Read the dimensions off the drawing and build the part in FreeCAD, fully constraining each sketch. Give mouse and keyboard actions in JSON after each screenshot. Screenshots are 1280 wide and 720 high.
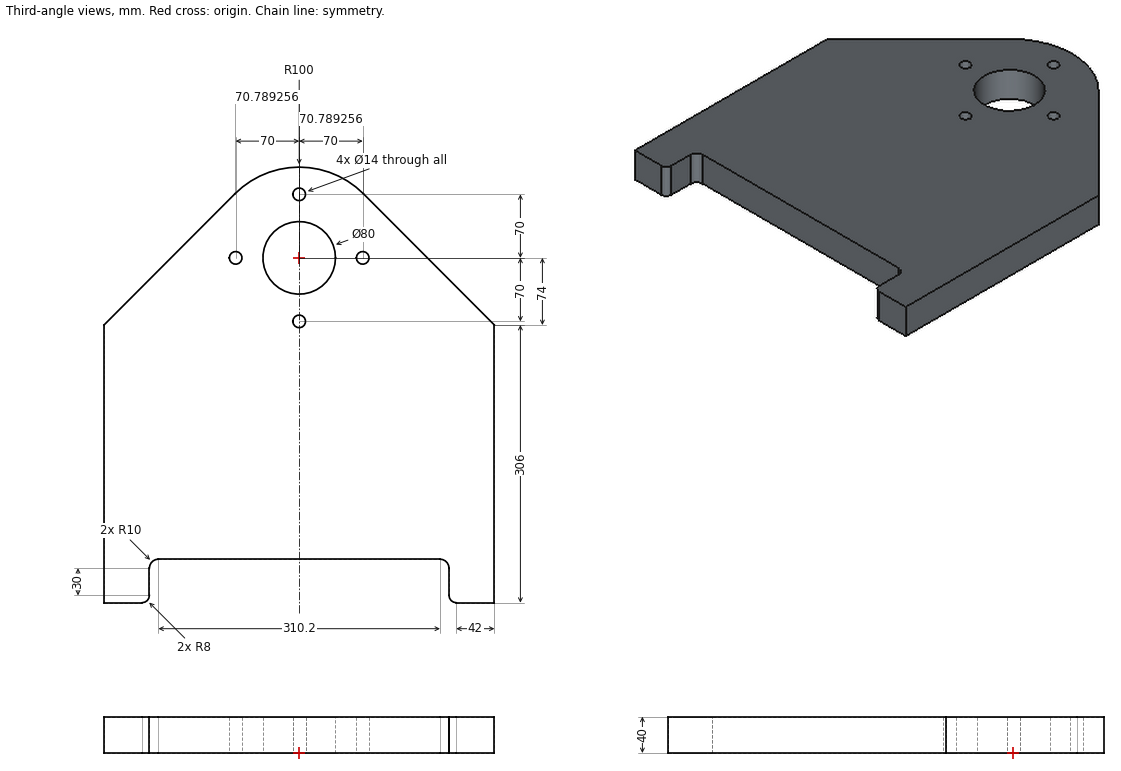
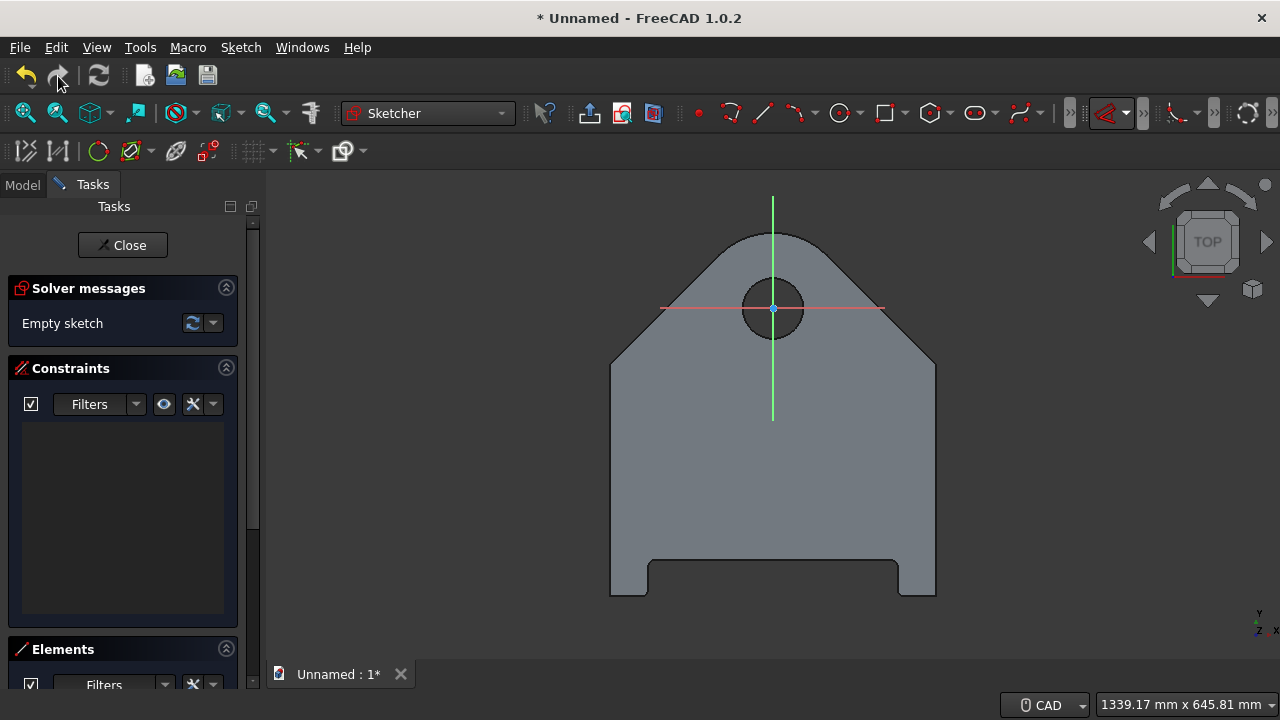
{"action": "scroll", "coordinate": [813, 247], "scroll_direction": "up", "scroll_amount": 5}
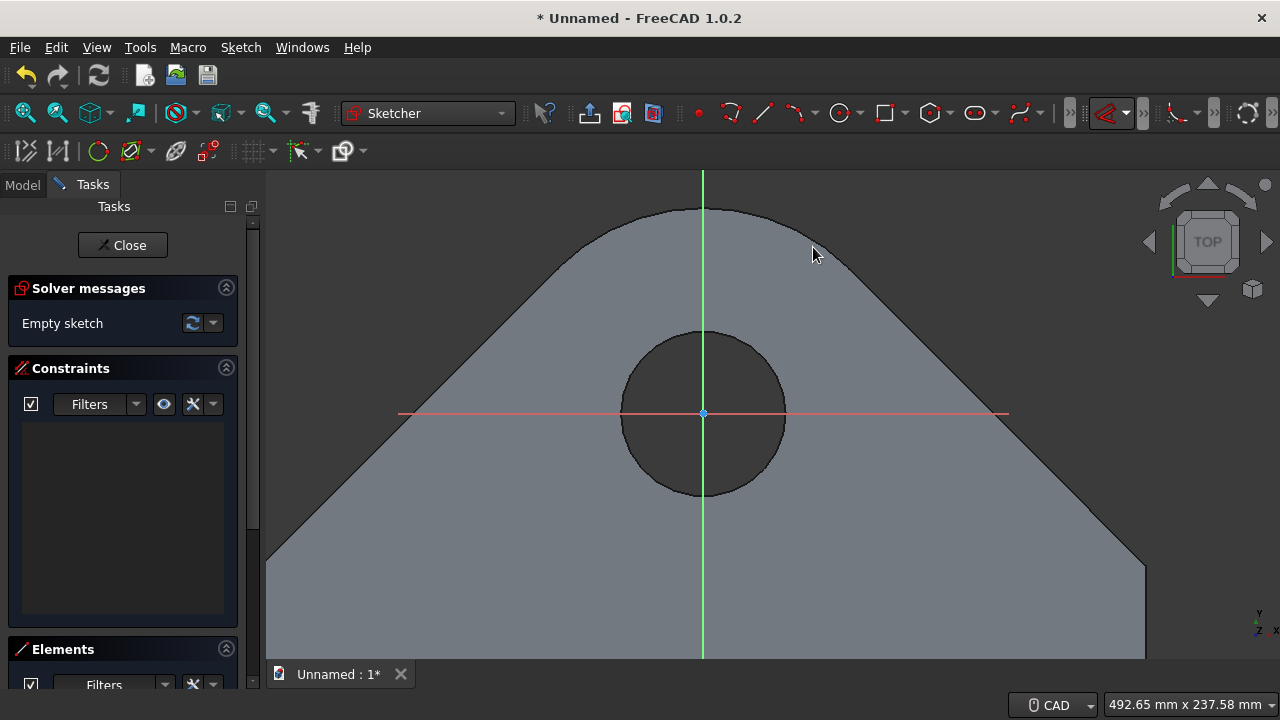
{"action": "key", "text": "g c"}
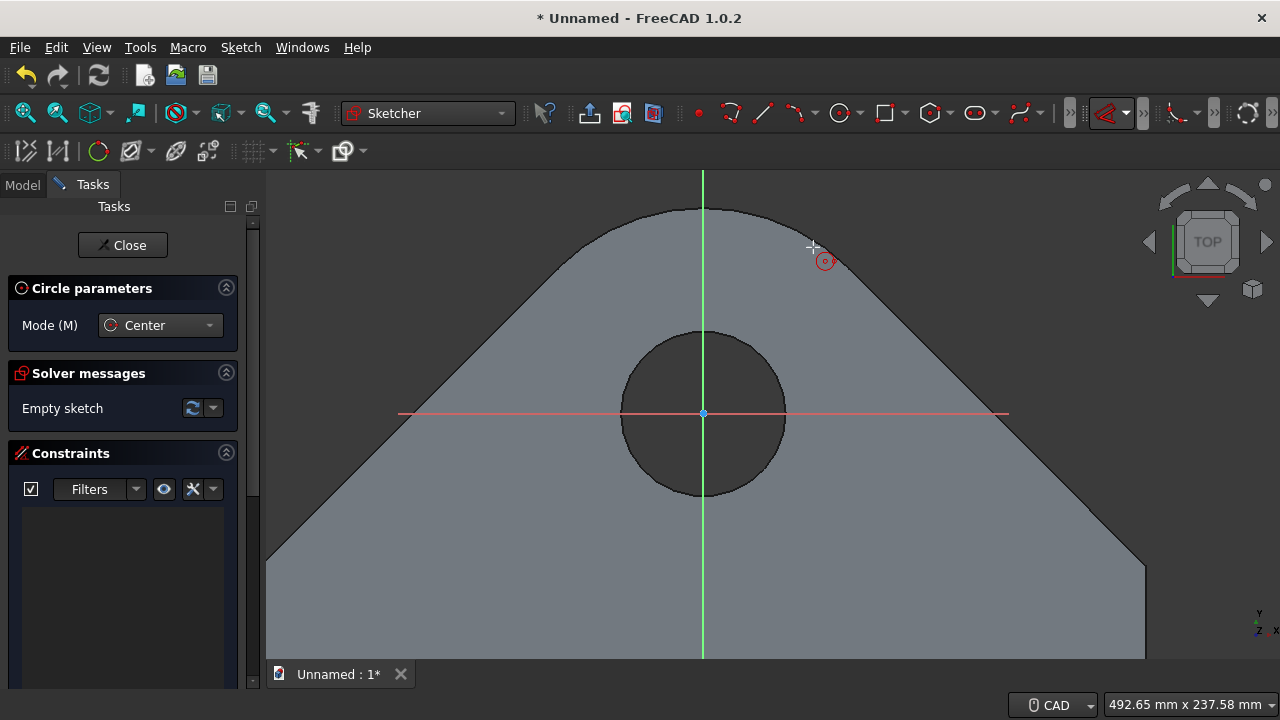
{"action": "scroll", "coordinate": [703, 270], "scroll_direction": "up", "scroll_amount": 3}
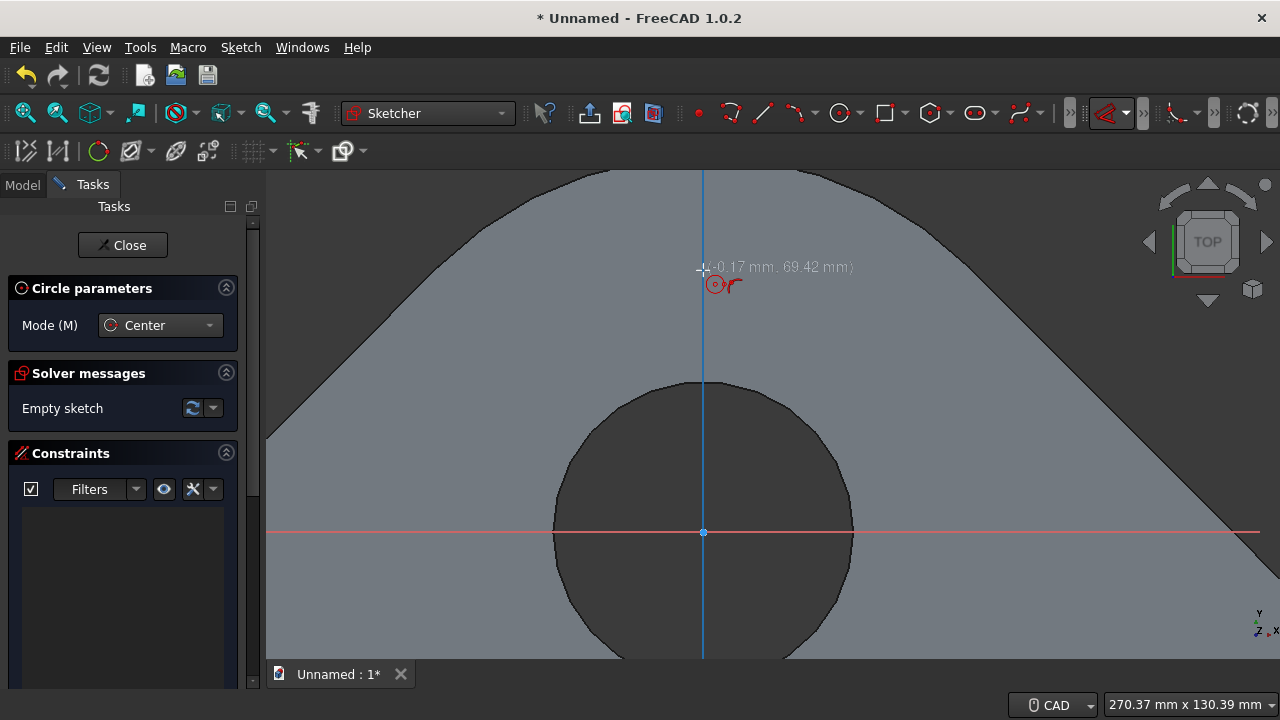
{"action": "left_click", "coordinate": [703, 269]}
{"action": "left_click", "coordinate": [722, 251]}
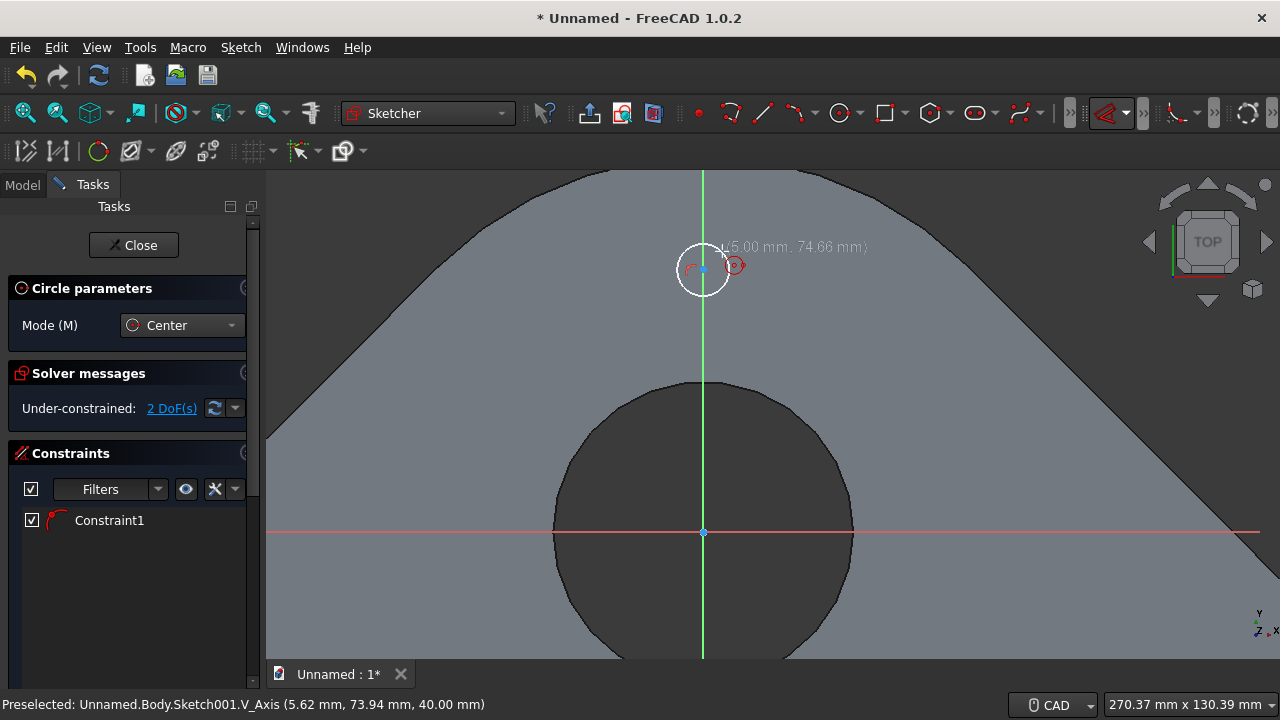
{"action": "left_click", "coordinate": [966, 532]}
{"action": "left_click", "coordinate": [984, 513]}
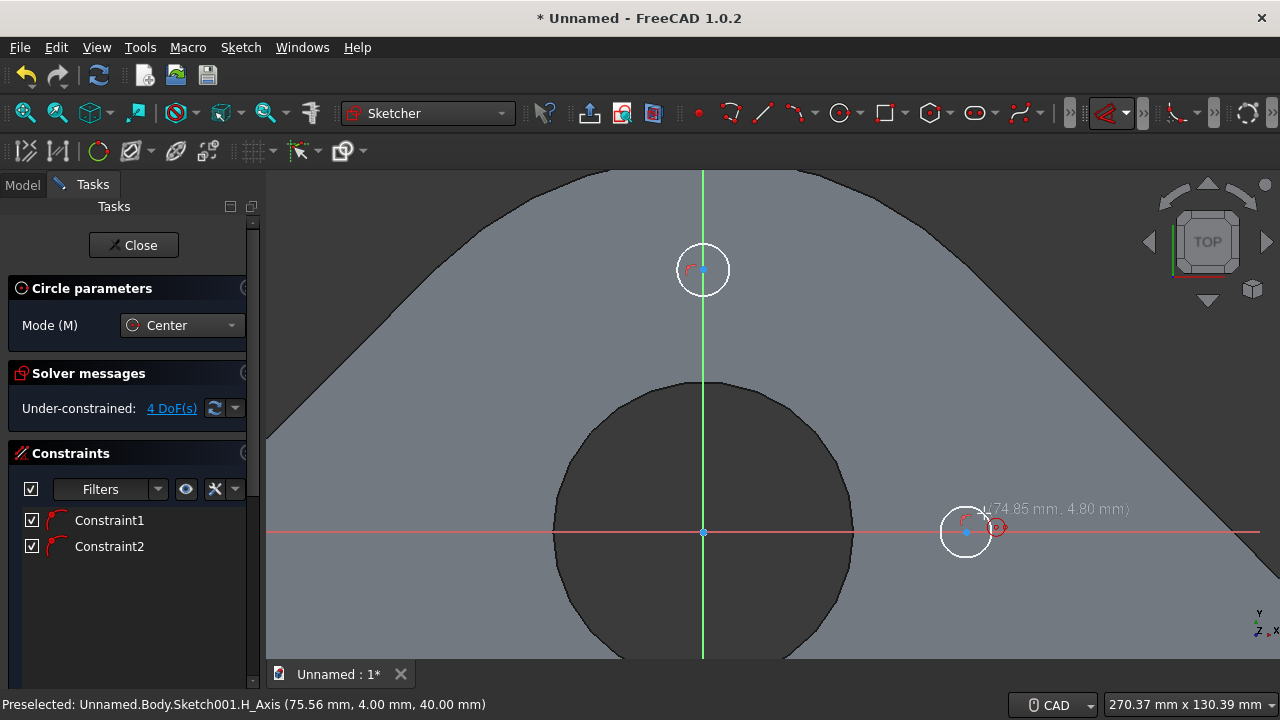
{"action": "scroll", "coordinate": [706, 272], "scroll_direction": "down", "scroll_amount": 3}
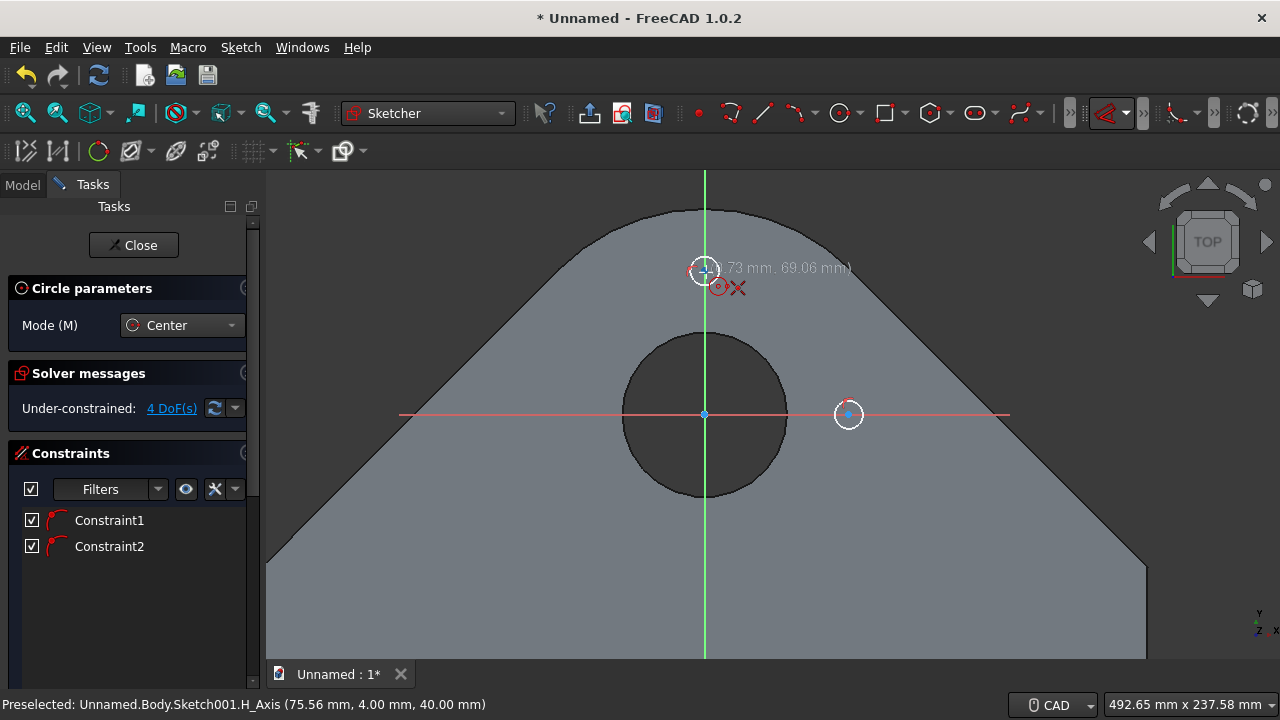
{"action": "scroll", "coordinate": [705, 559], "scroll_direction": "up", "scroll_amount": 3}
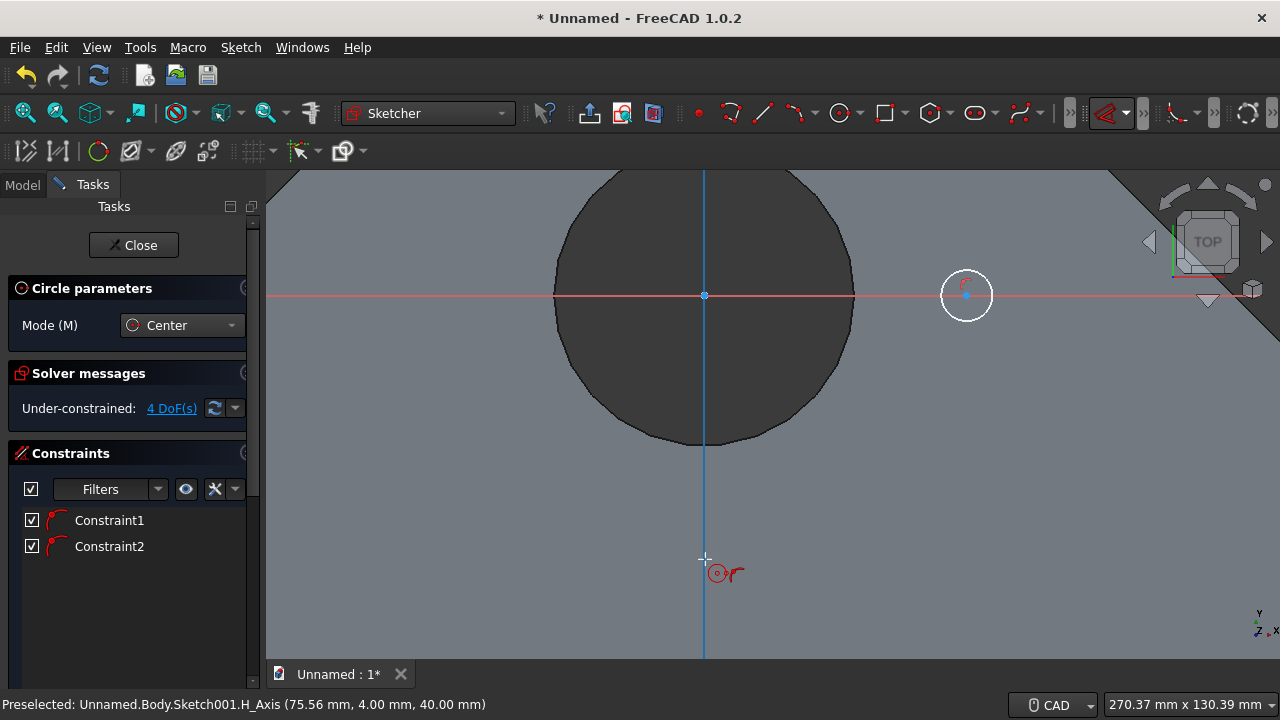
{"action": "left_click", "coordinate": [704, 558]}
{"action": "left_click", "coordinate": [723, 540]}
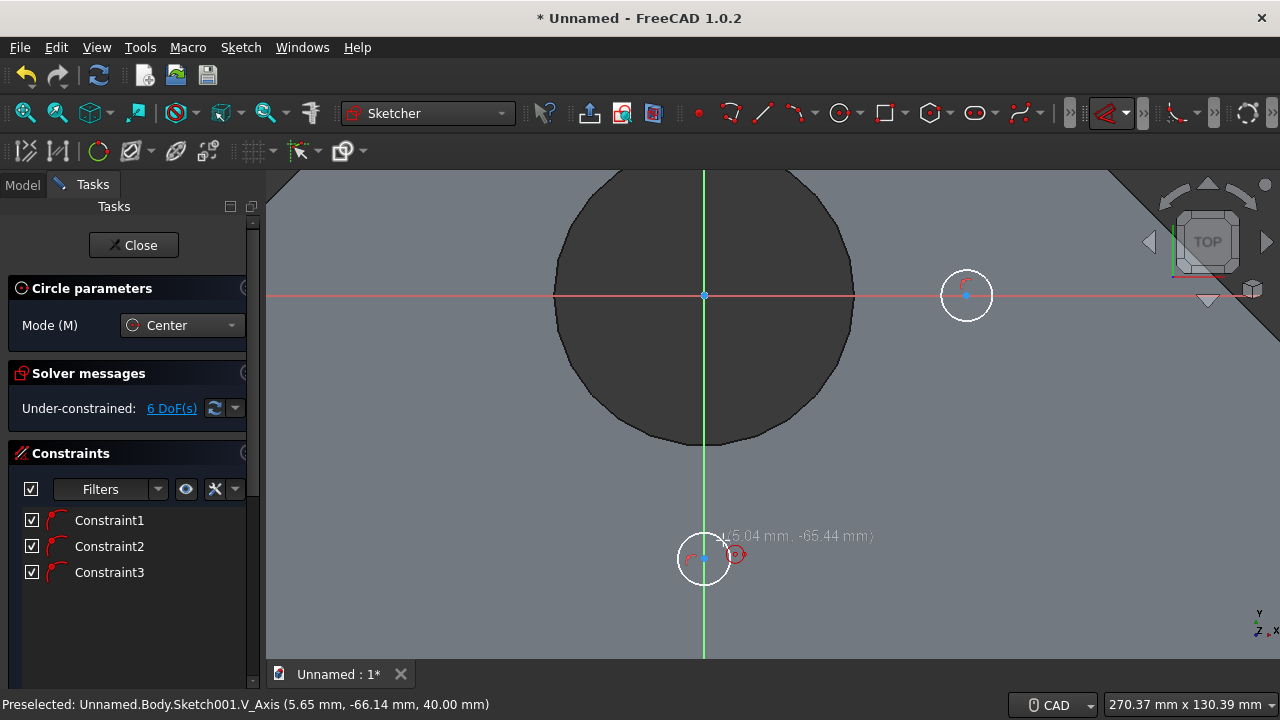
{"action": "left_click", "coordinate": [442, 296]}
{"action": "left_click", "coordinate": [460, 277]}
{"action": "key", "text": "Escape"}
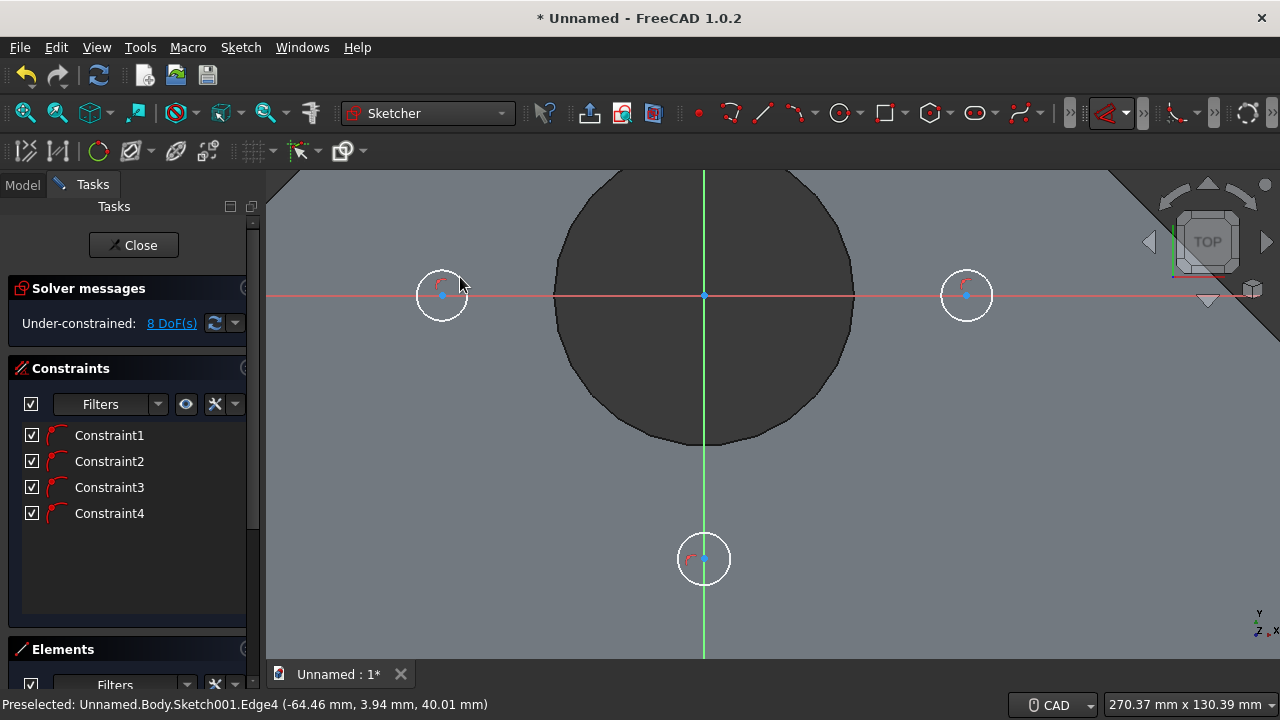
{"action": "scroll", "coordinate": [705, 559], "scroll_direction": "down", "scroll_amount": 3}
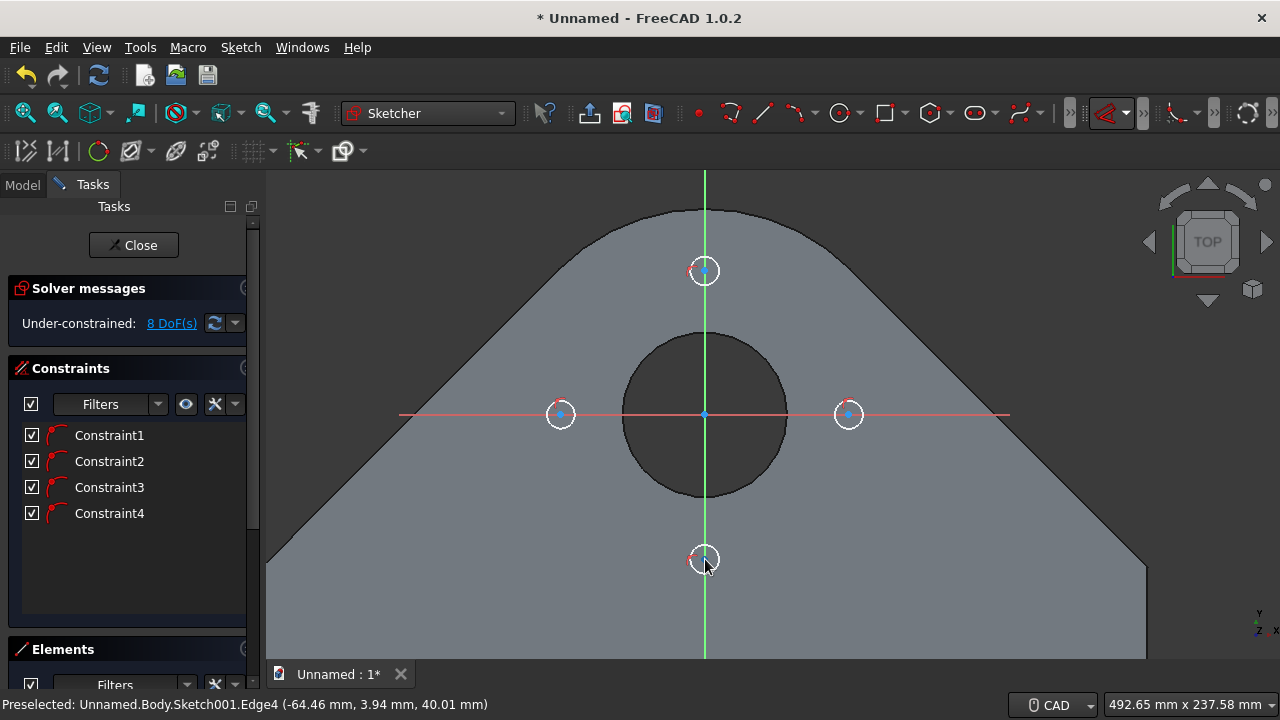
{"action": "scroll", "coordinate": [715, 261], "scroll_direction": "up", "scroll_amount": 2}